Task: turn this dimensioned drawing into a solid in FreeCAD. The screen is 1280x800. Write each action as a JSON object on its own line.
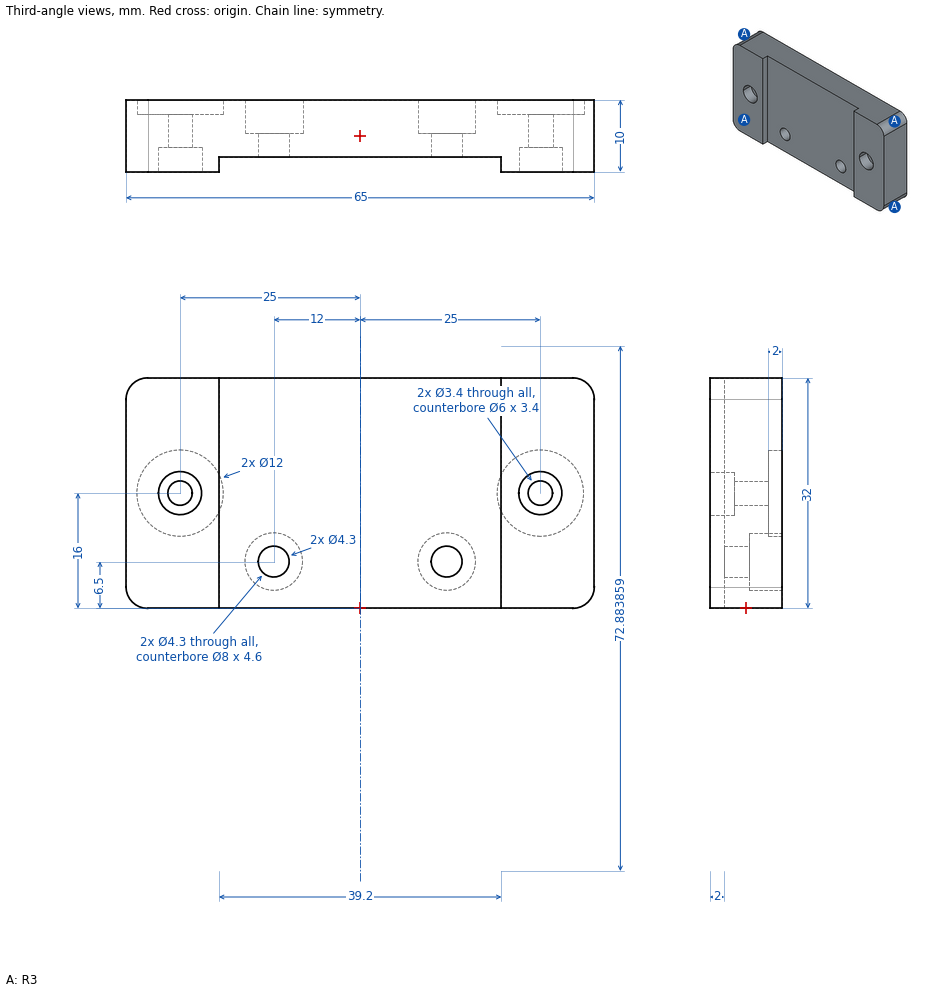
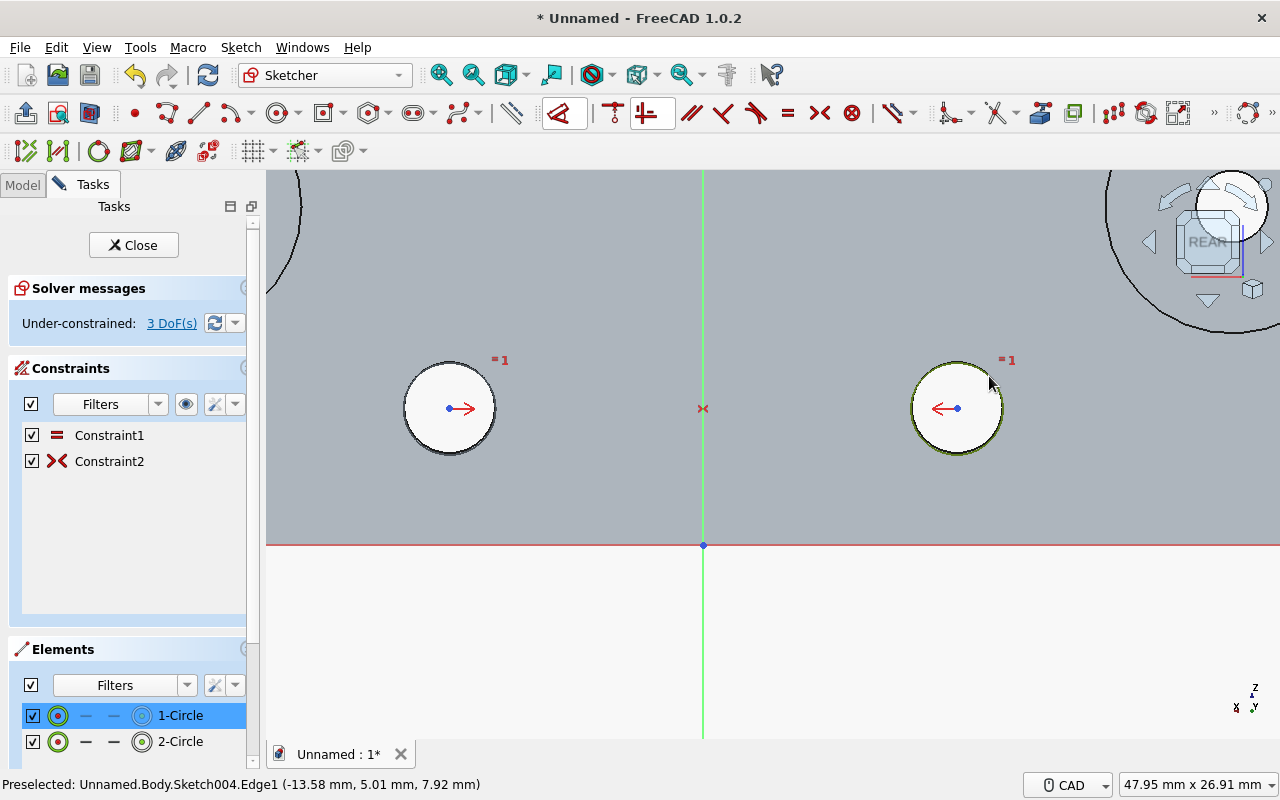
{"action": "left_click", "coordinate": [582, 114]}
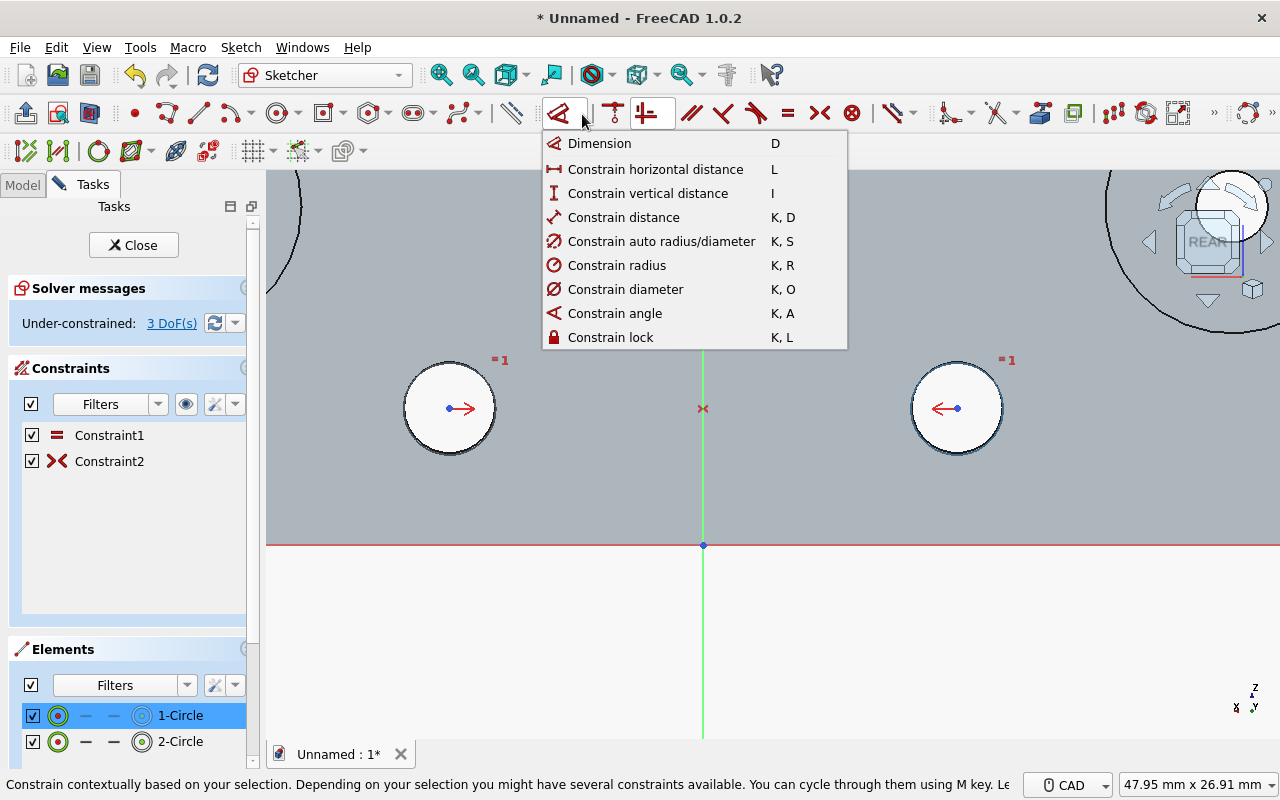
{"action": "left_click", "coordinate": [695, 289]}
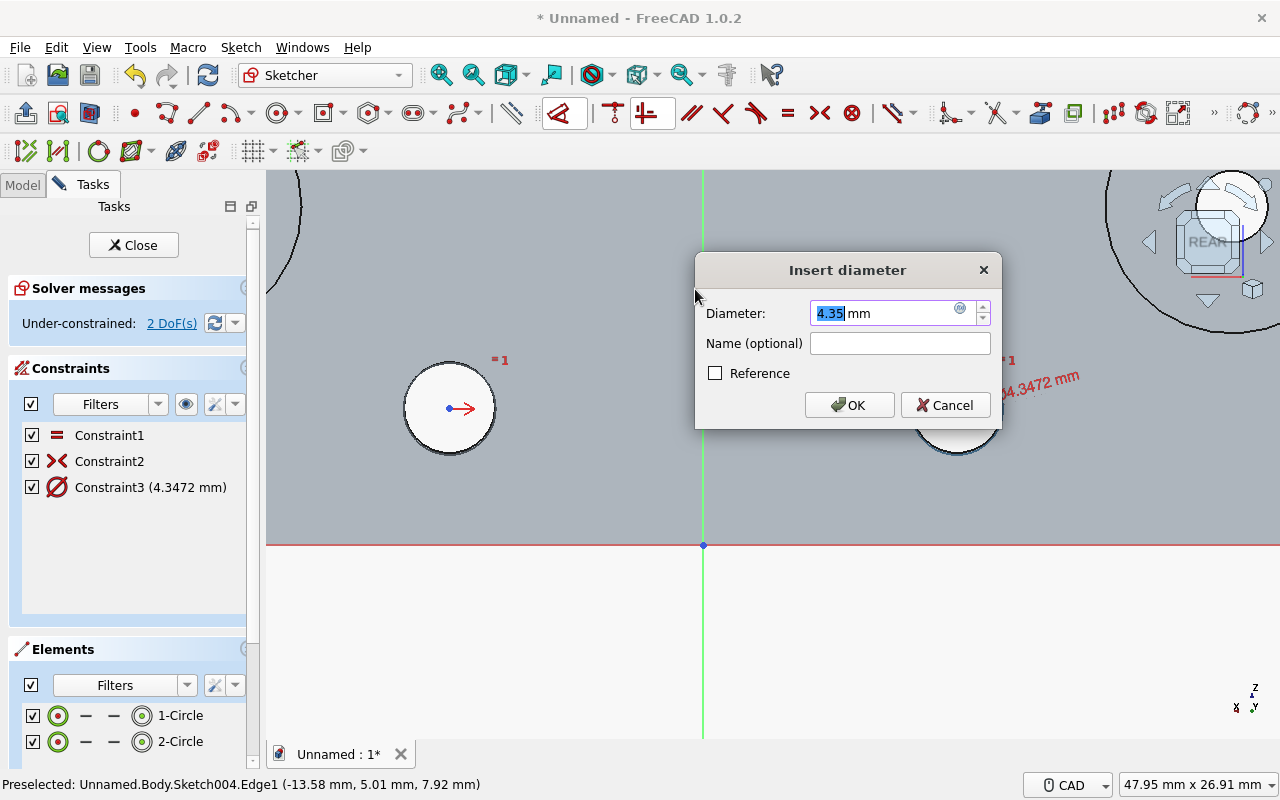
{"action": "type", "text": "4.3"}
{"action": "key", "text": "Return"}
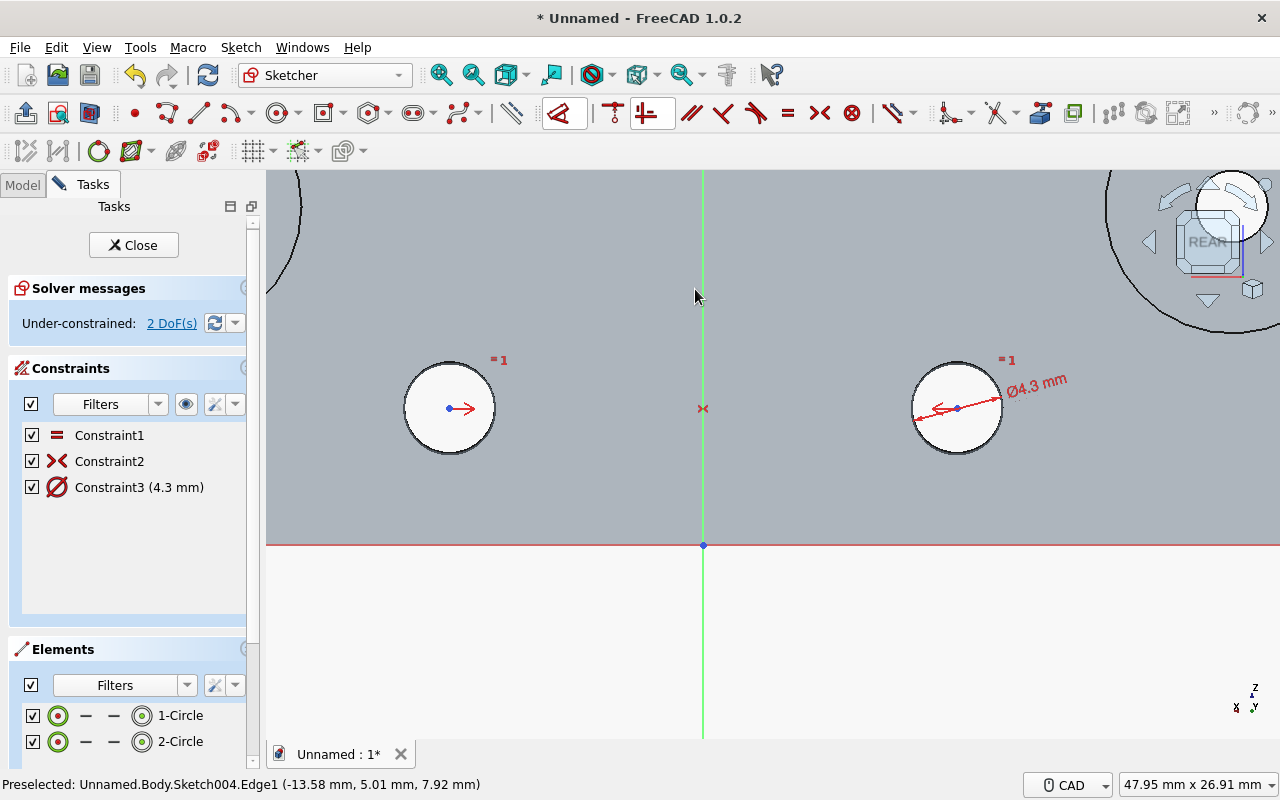
{"action": "left_click", "coordinate": [957, 409]}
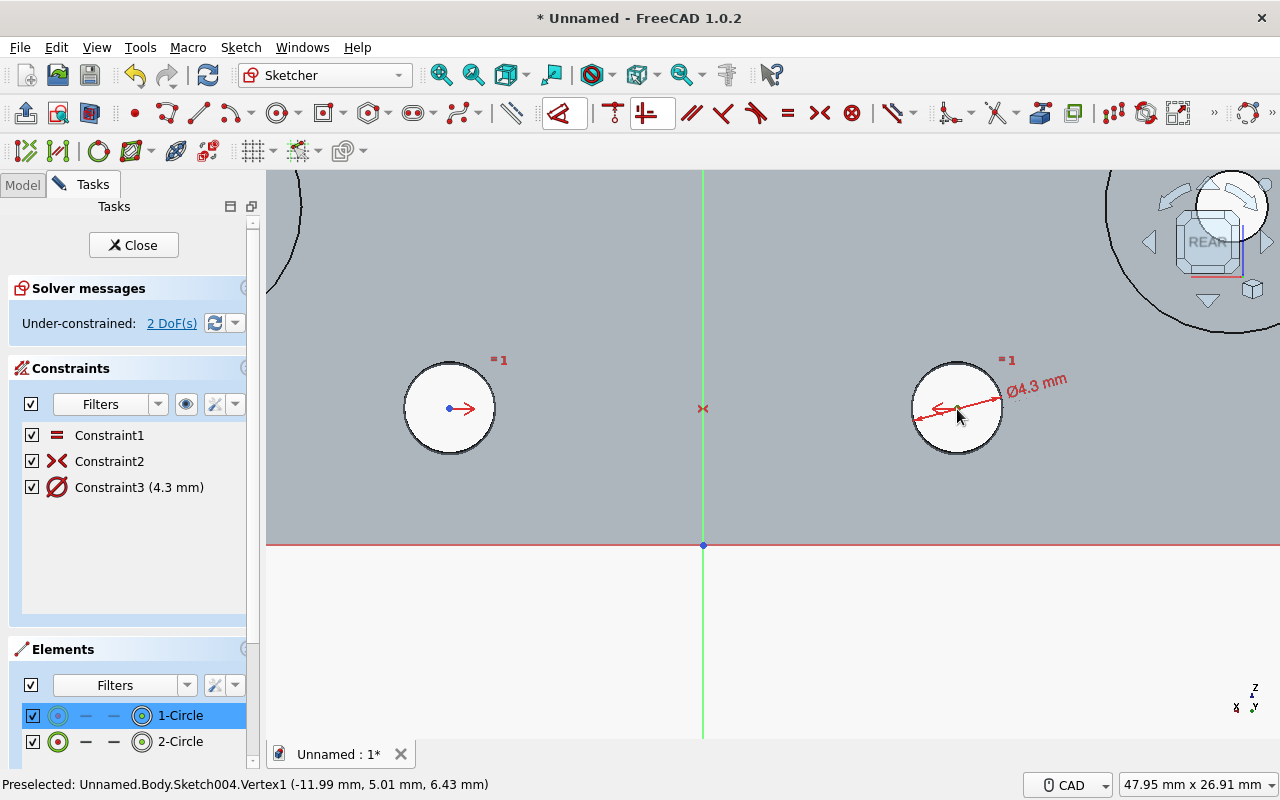
{"action": "key", "text": "l"}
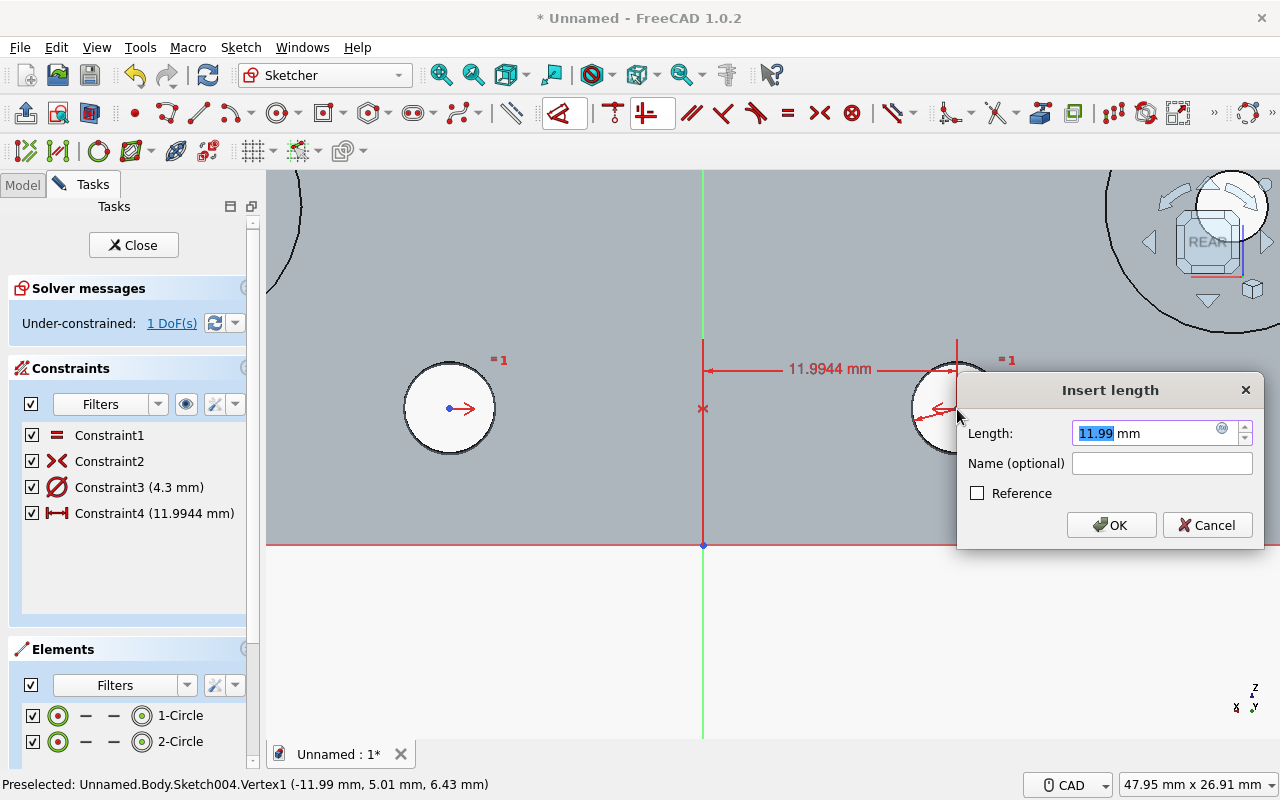
{"action": "type", "text": "12"}
{"action": "key", "text": "Return"}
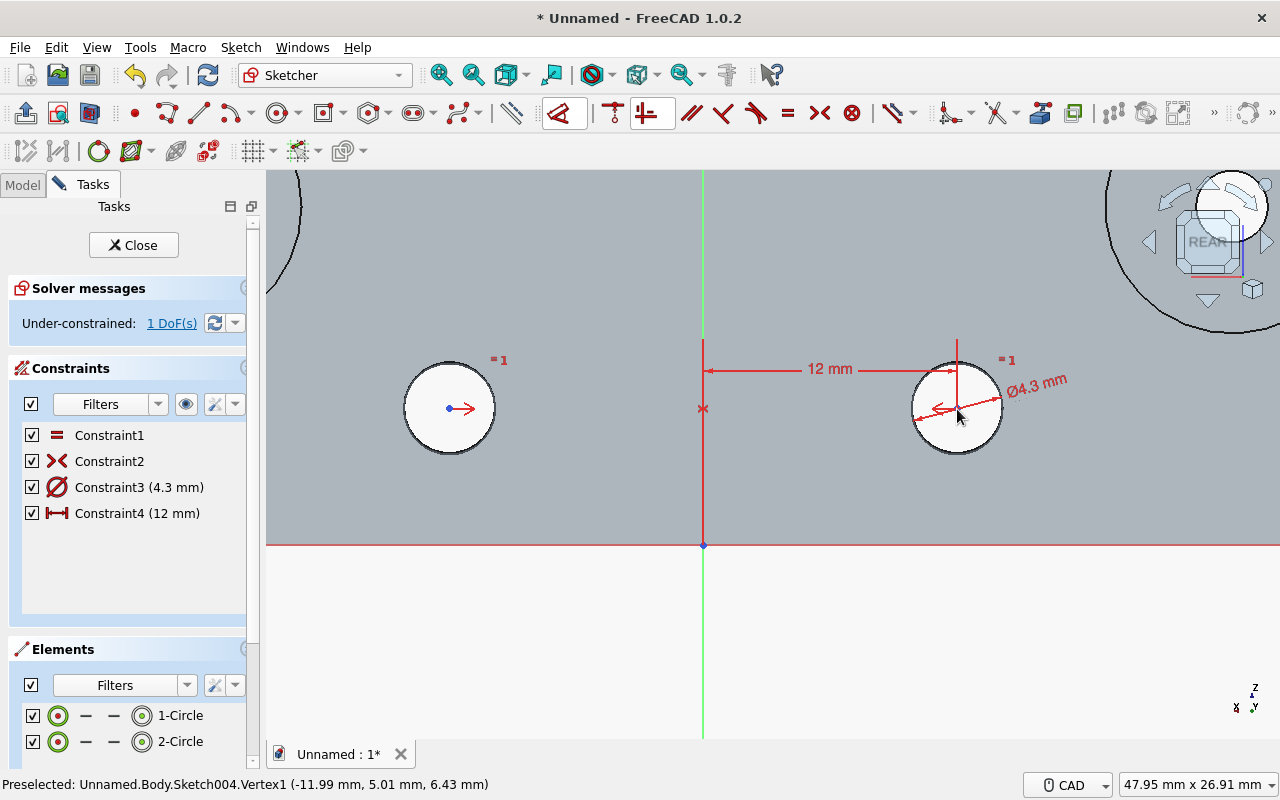
{"action": "left_click", "coordinate": [957, 409]}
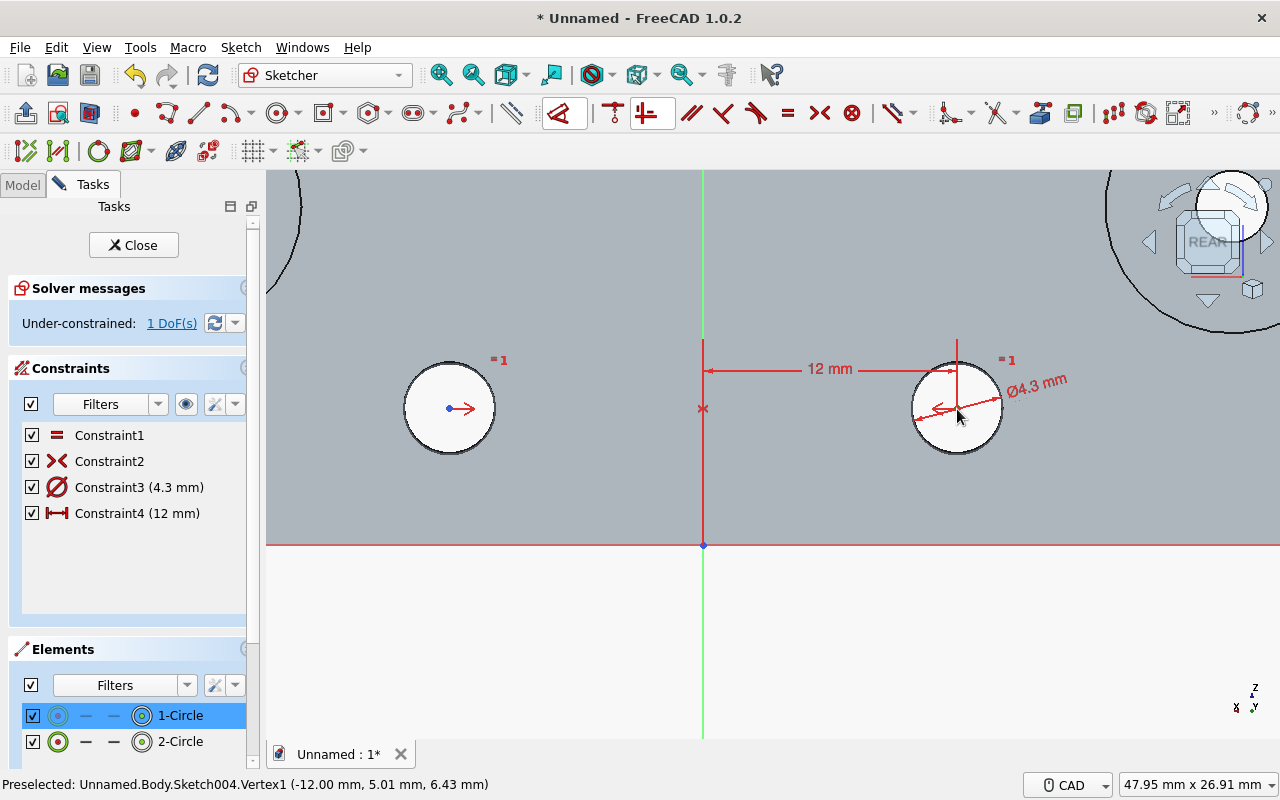
{"action": "key", "text": "i"}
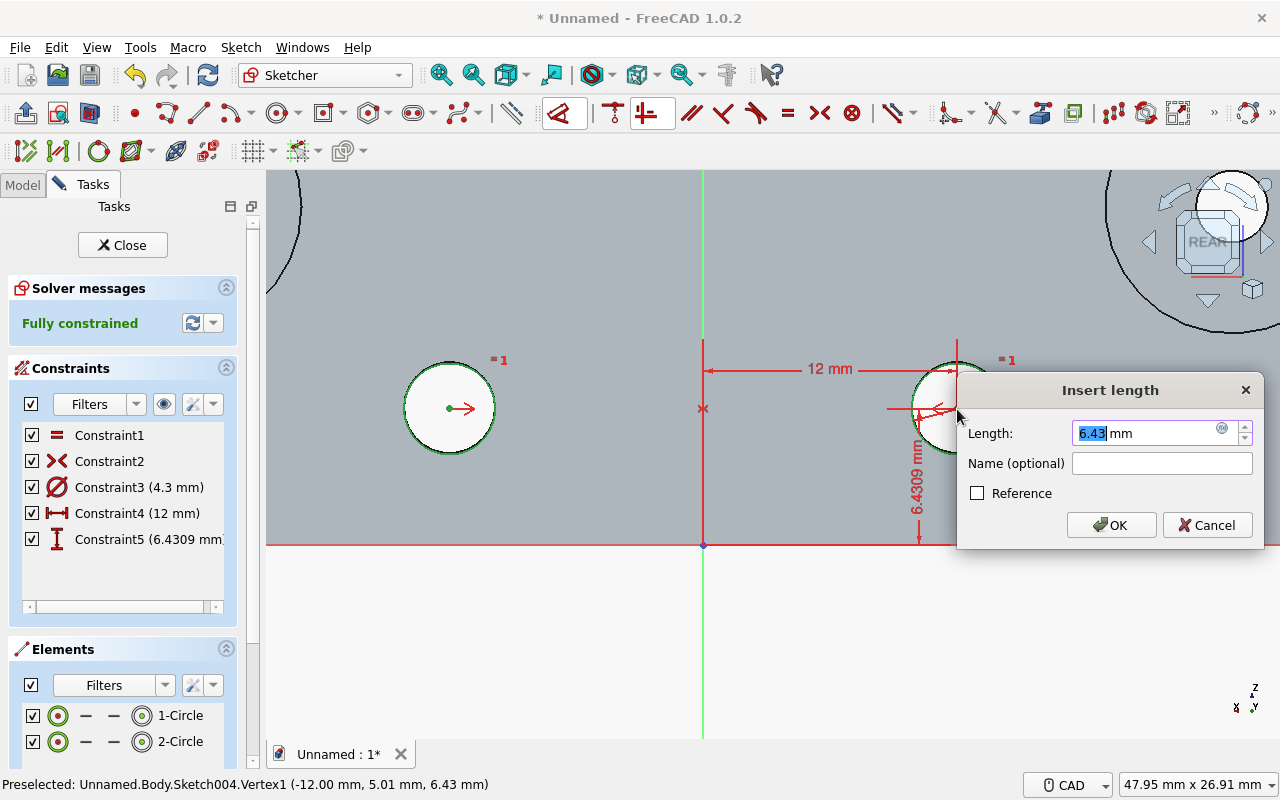
{"action": "type", "text": "6.5"}
{"action": "key", "text": "Return"}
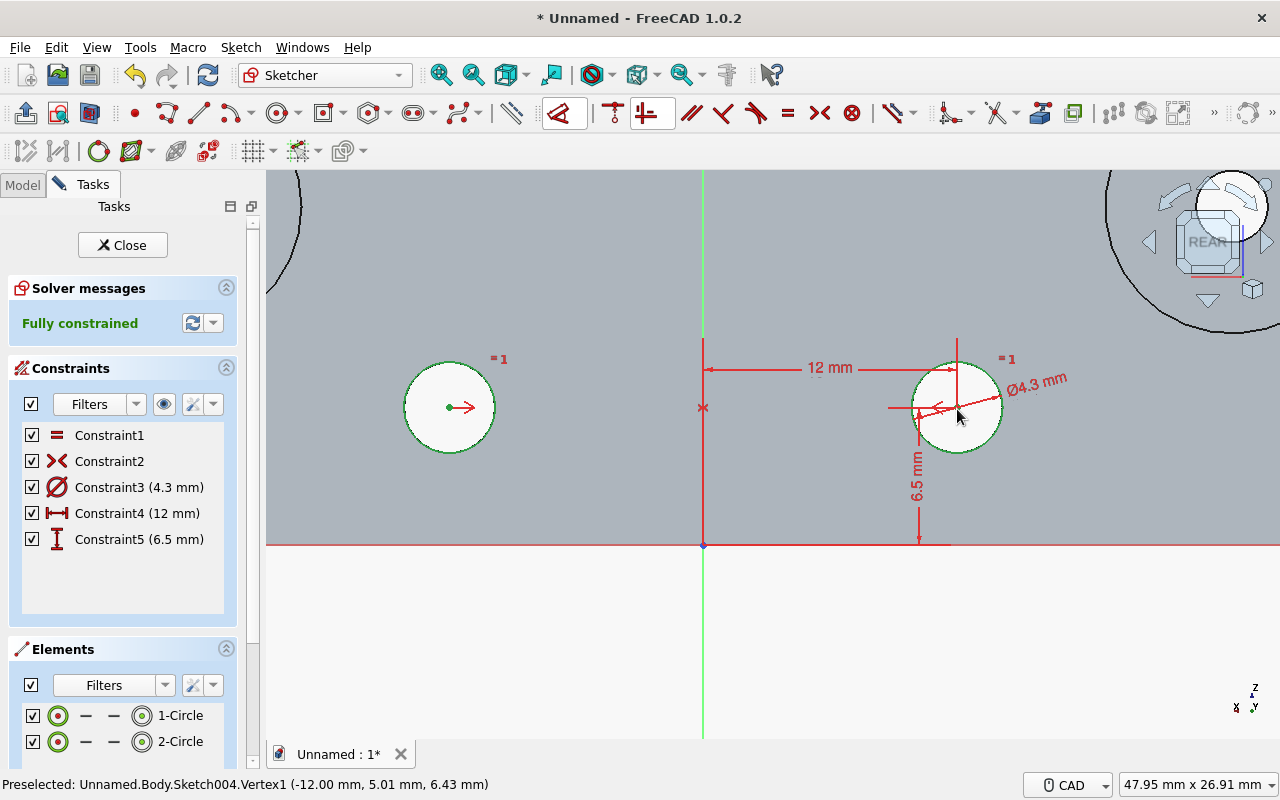
{"action": "left_click", "coordinate": [123, 245]}